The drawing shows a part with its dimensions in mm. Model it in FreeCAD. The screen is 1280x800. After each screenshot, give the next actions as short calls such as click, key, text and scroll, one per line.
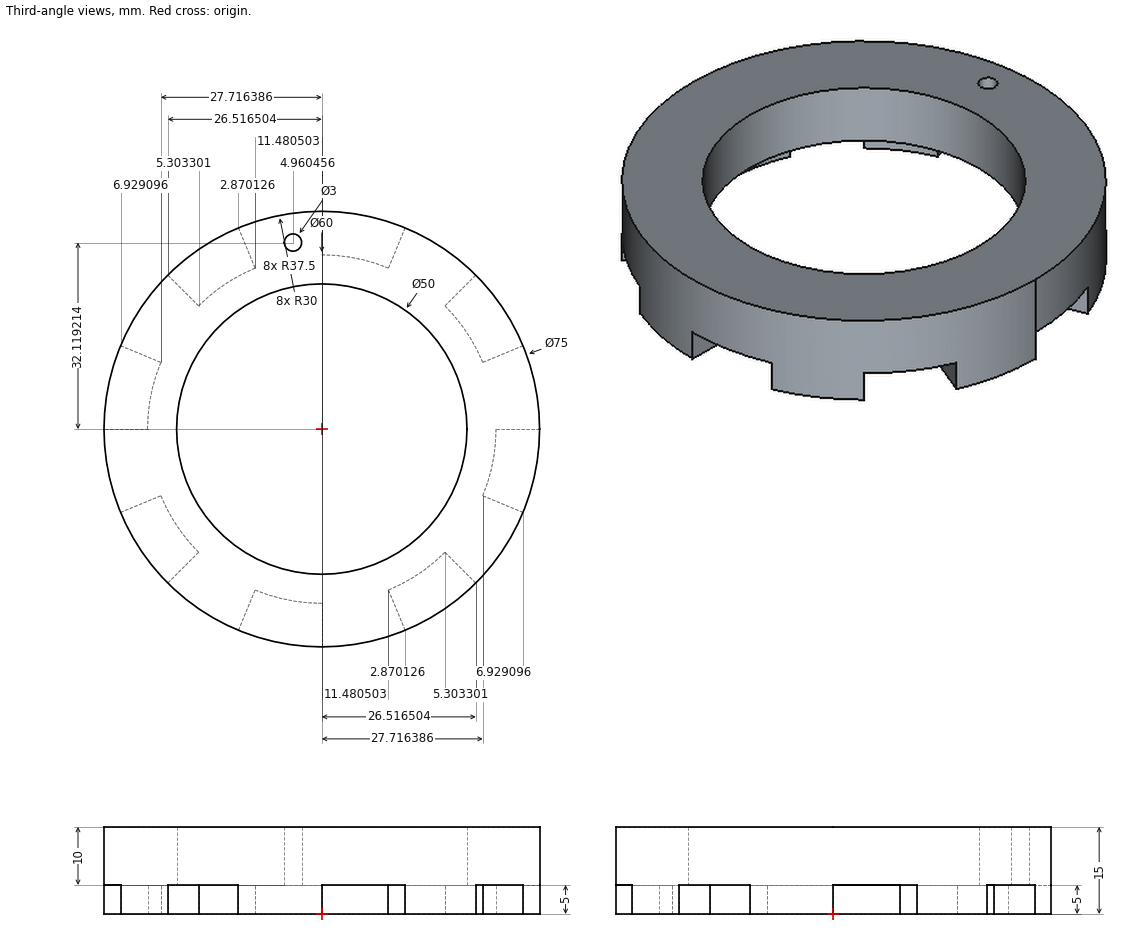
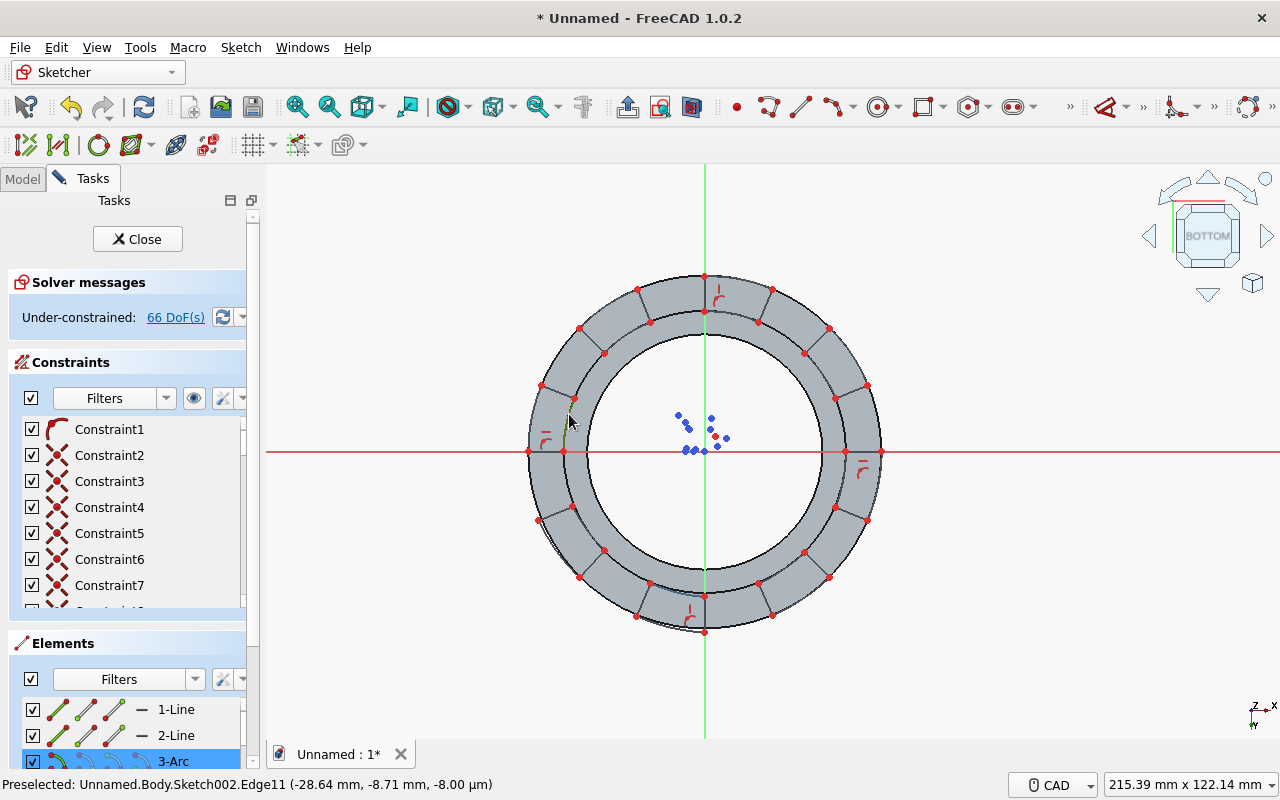
key(c)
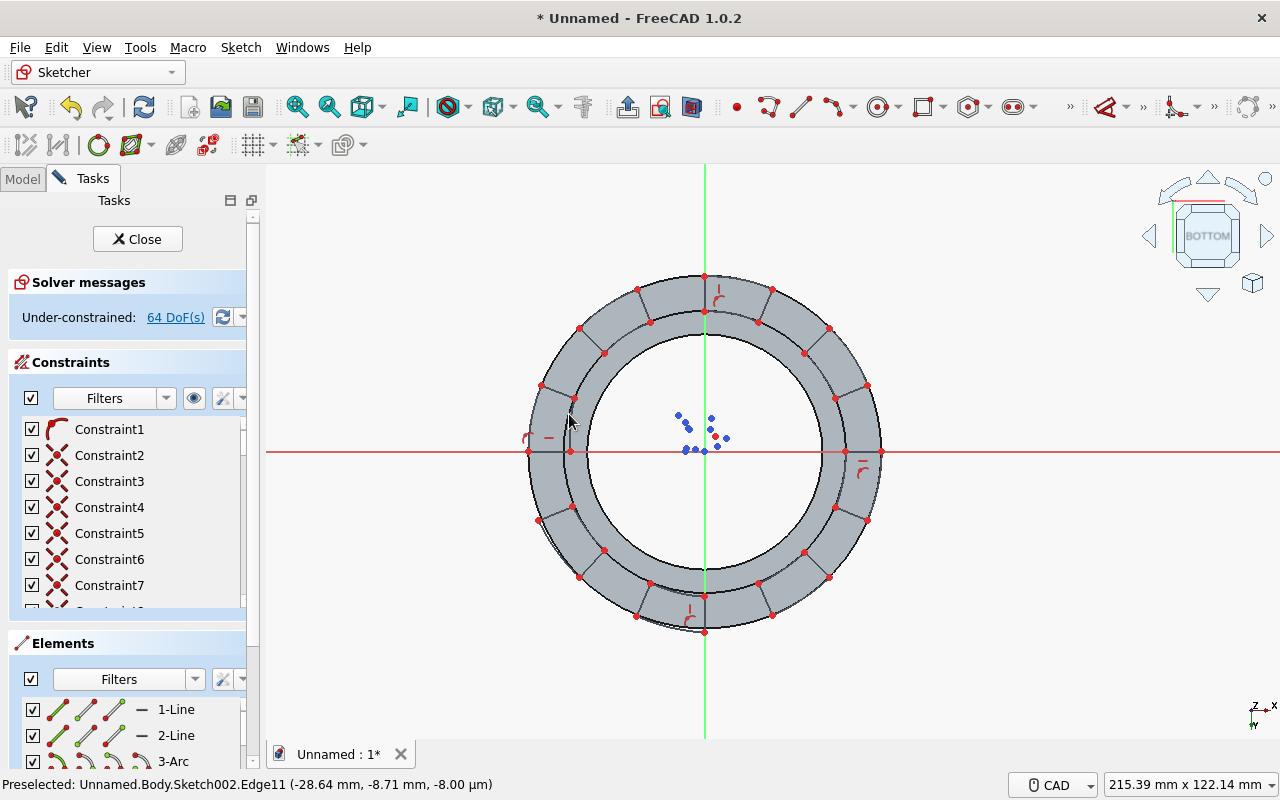
click(666, 589)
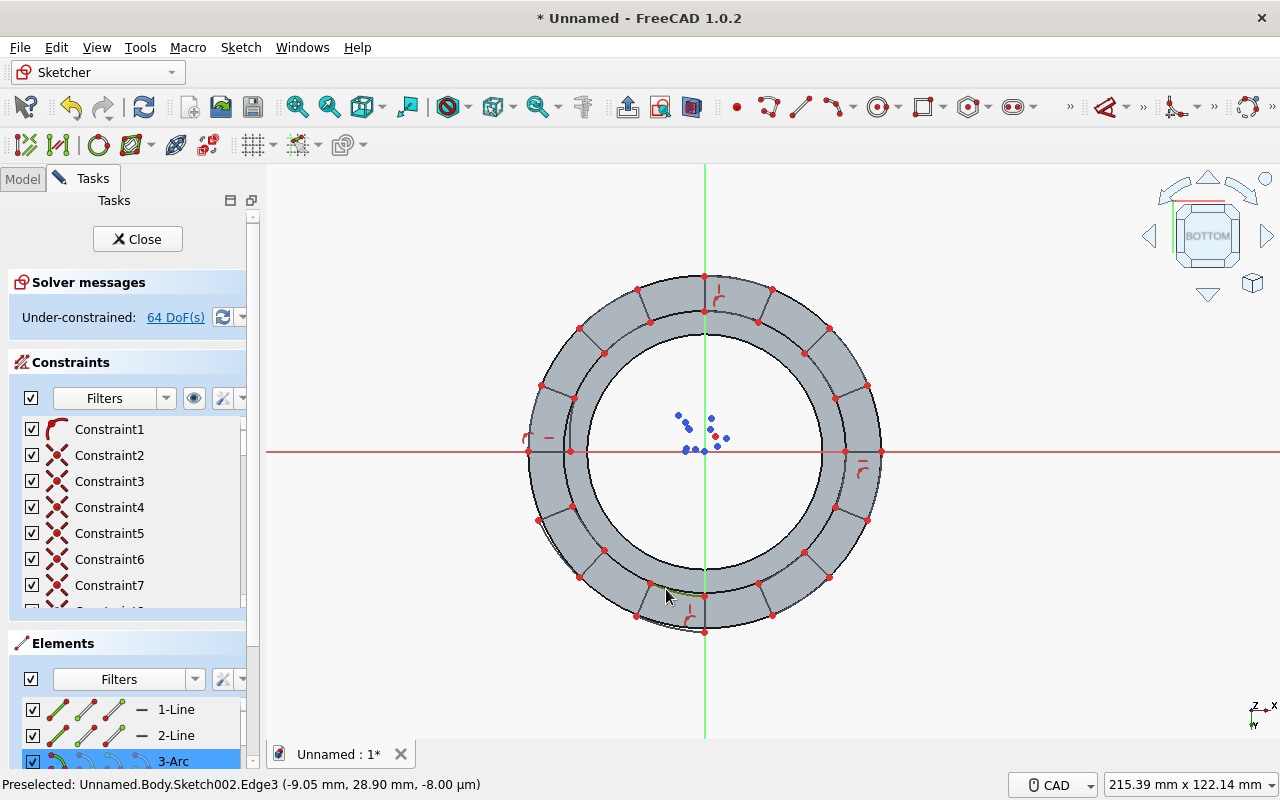
click(535, 405)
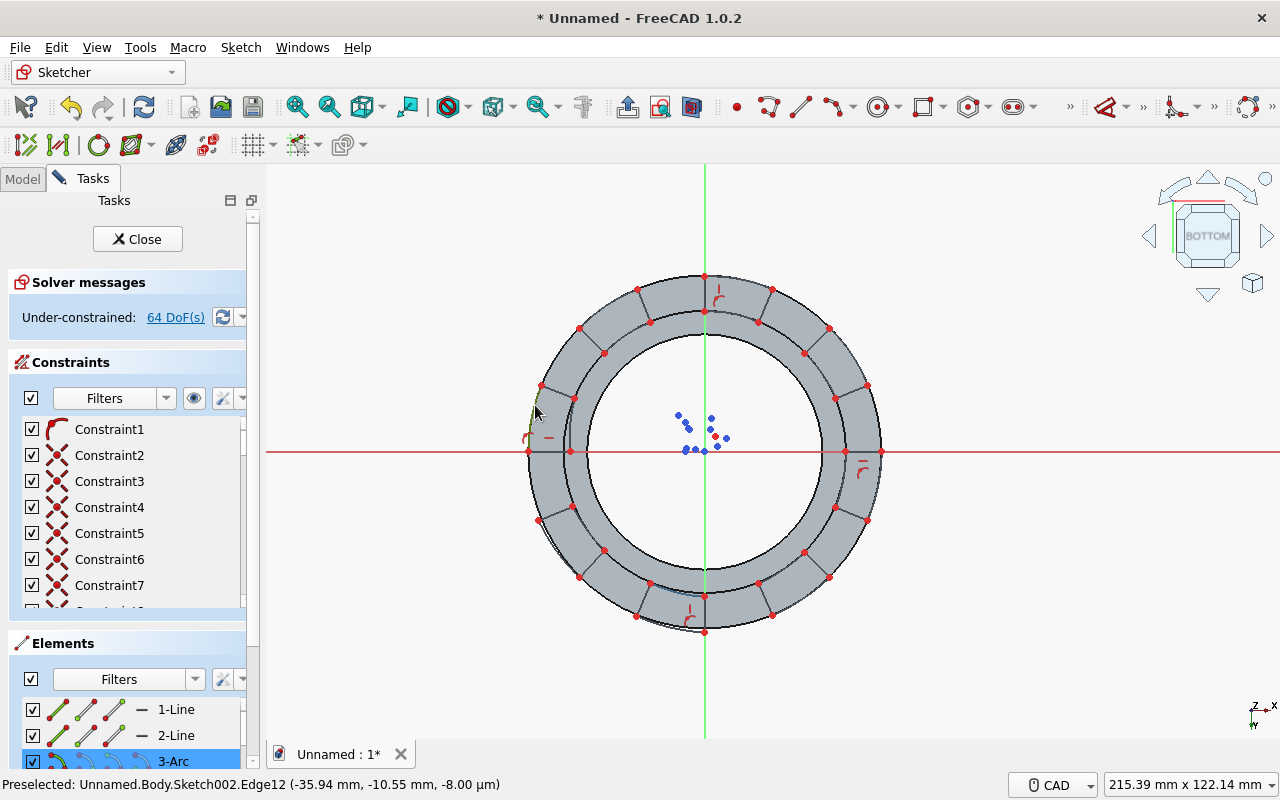
key(c)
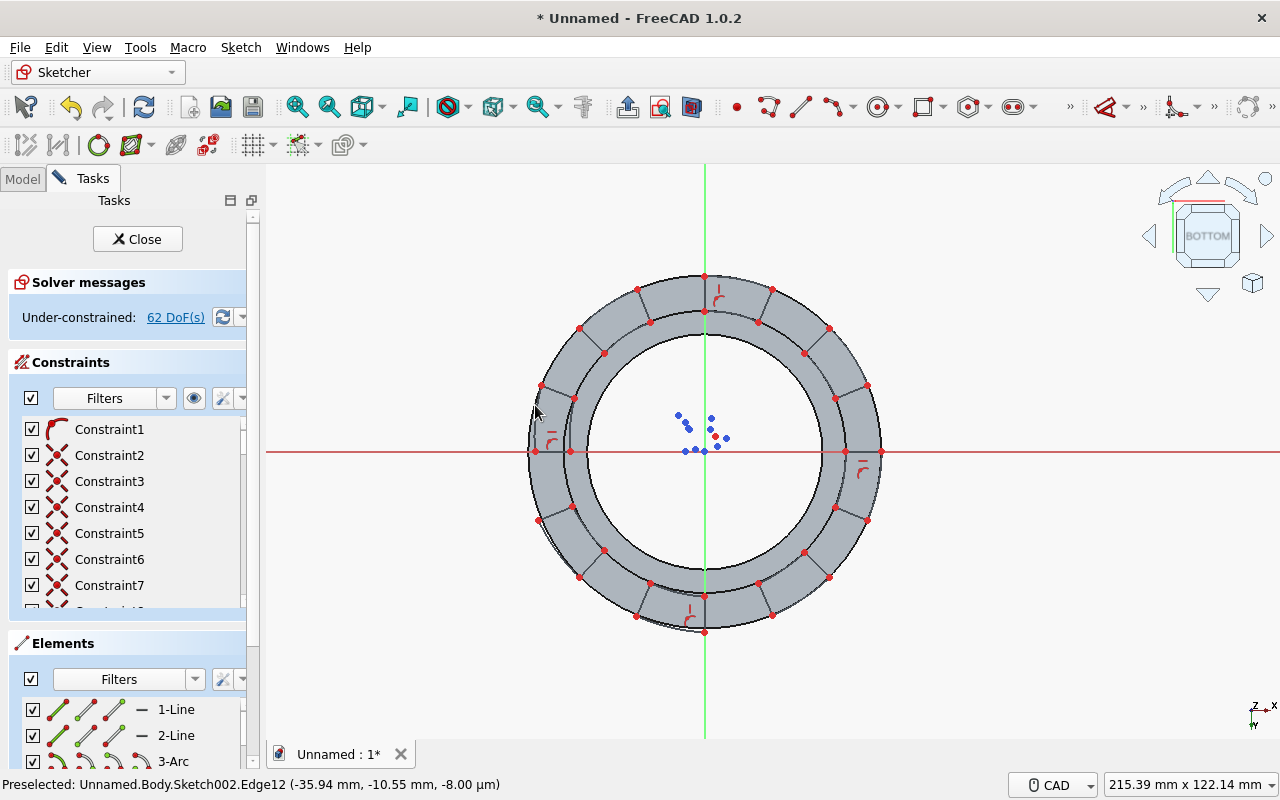
click(666, 589)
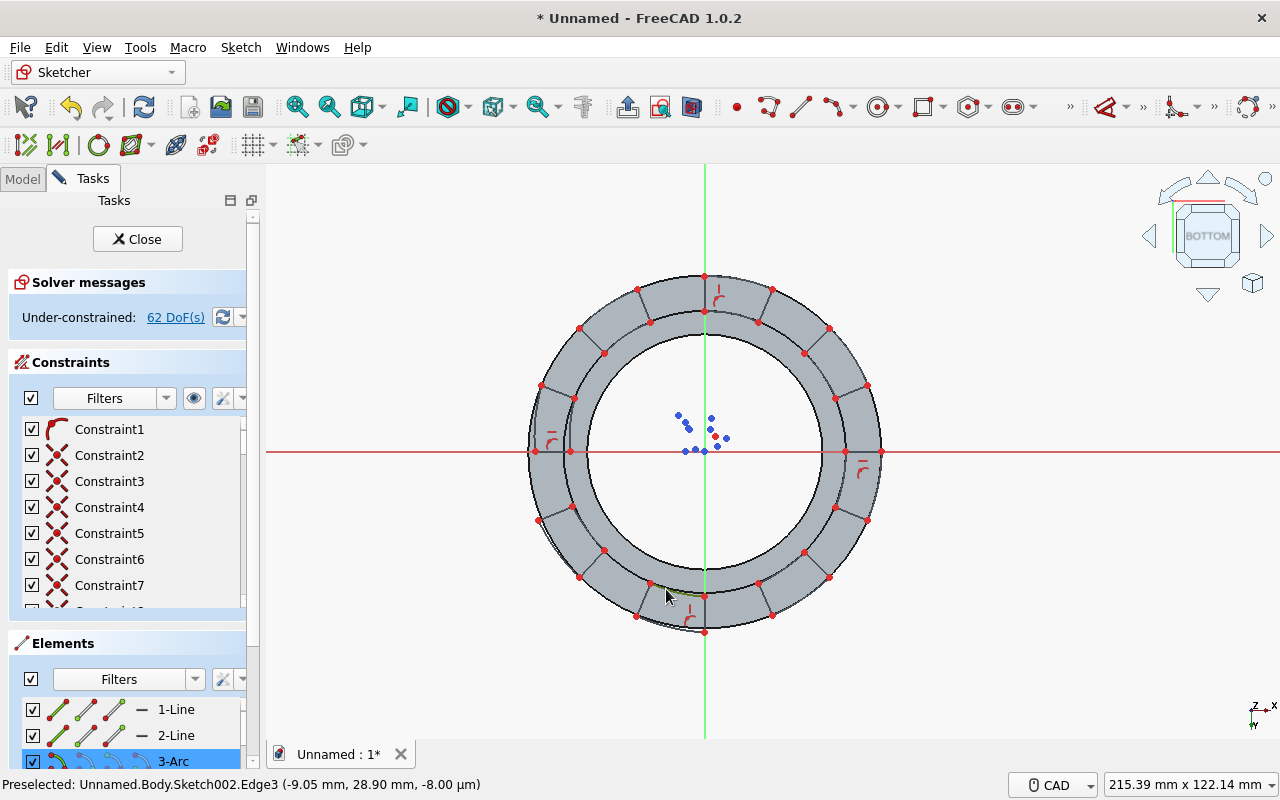
click(635, 329)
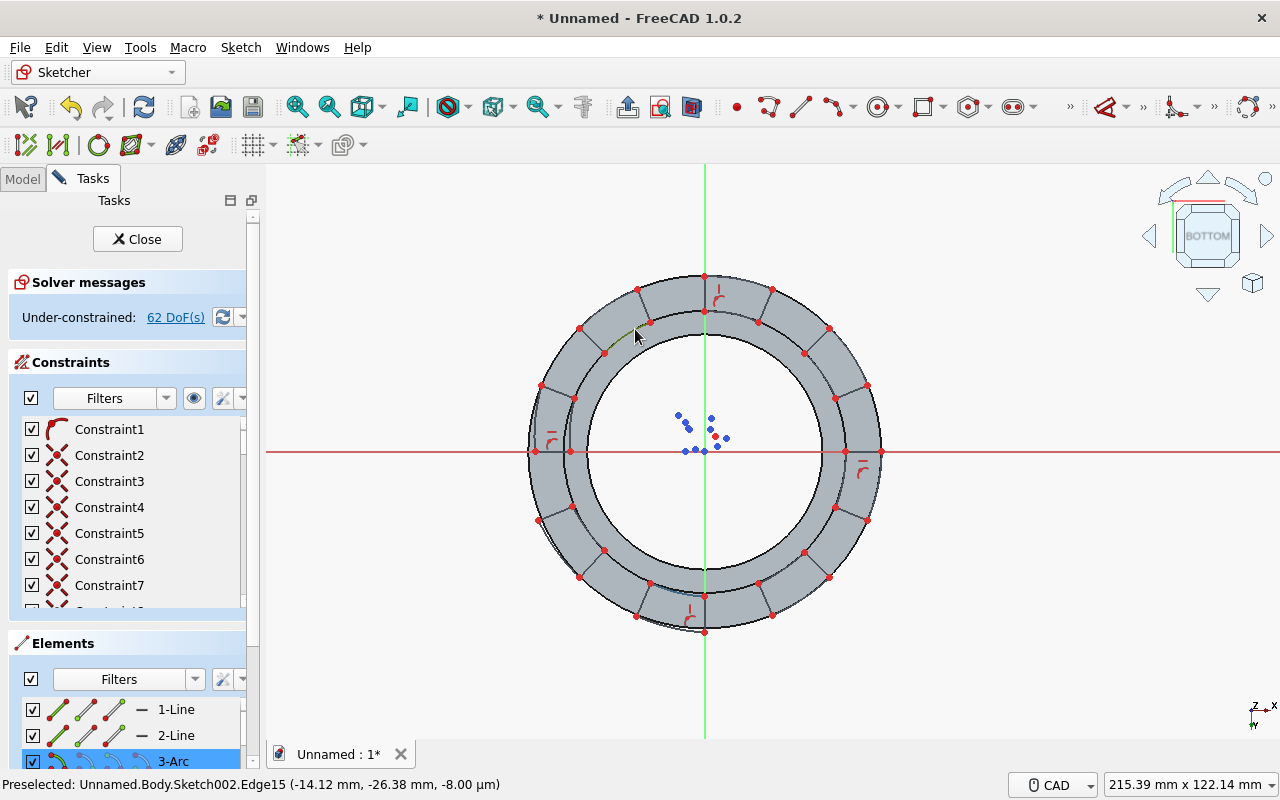
key(c)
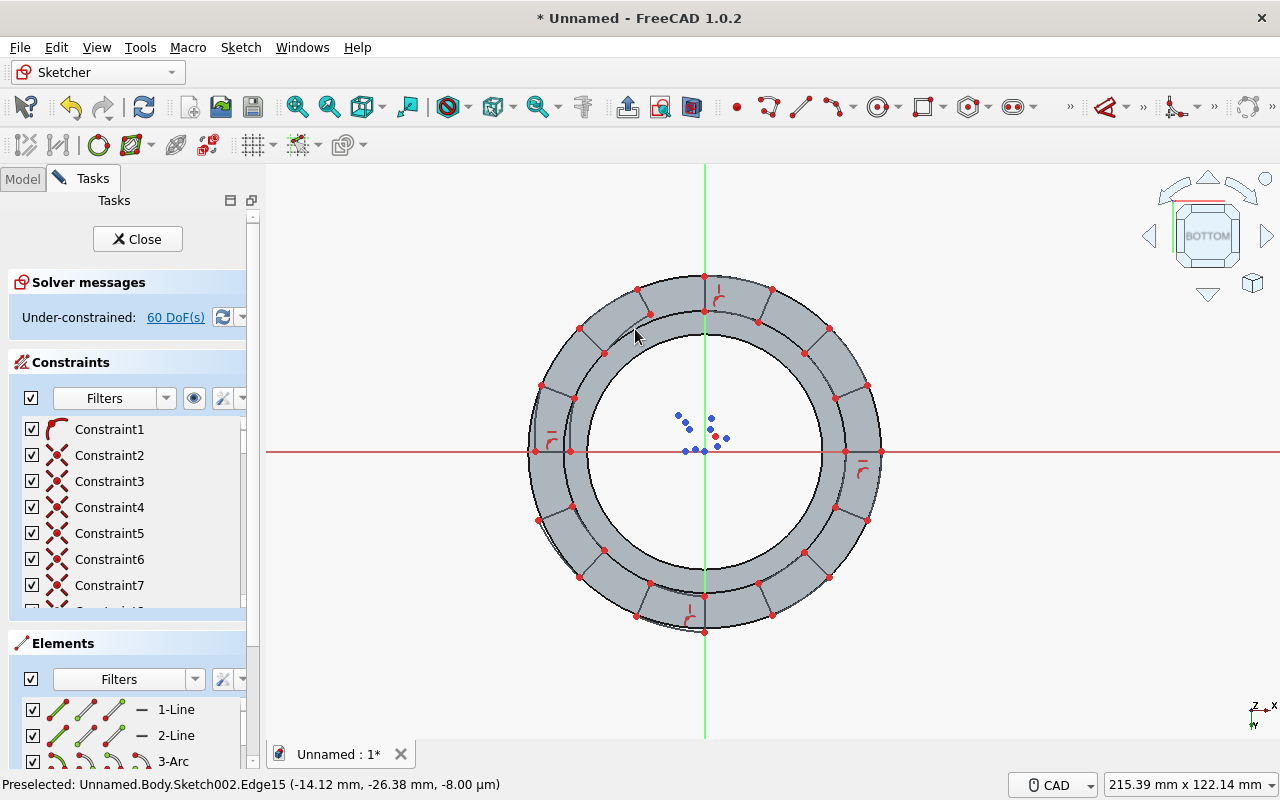
click(666, 589)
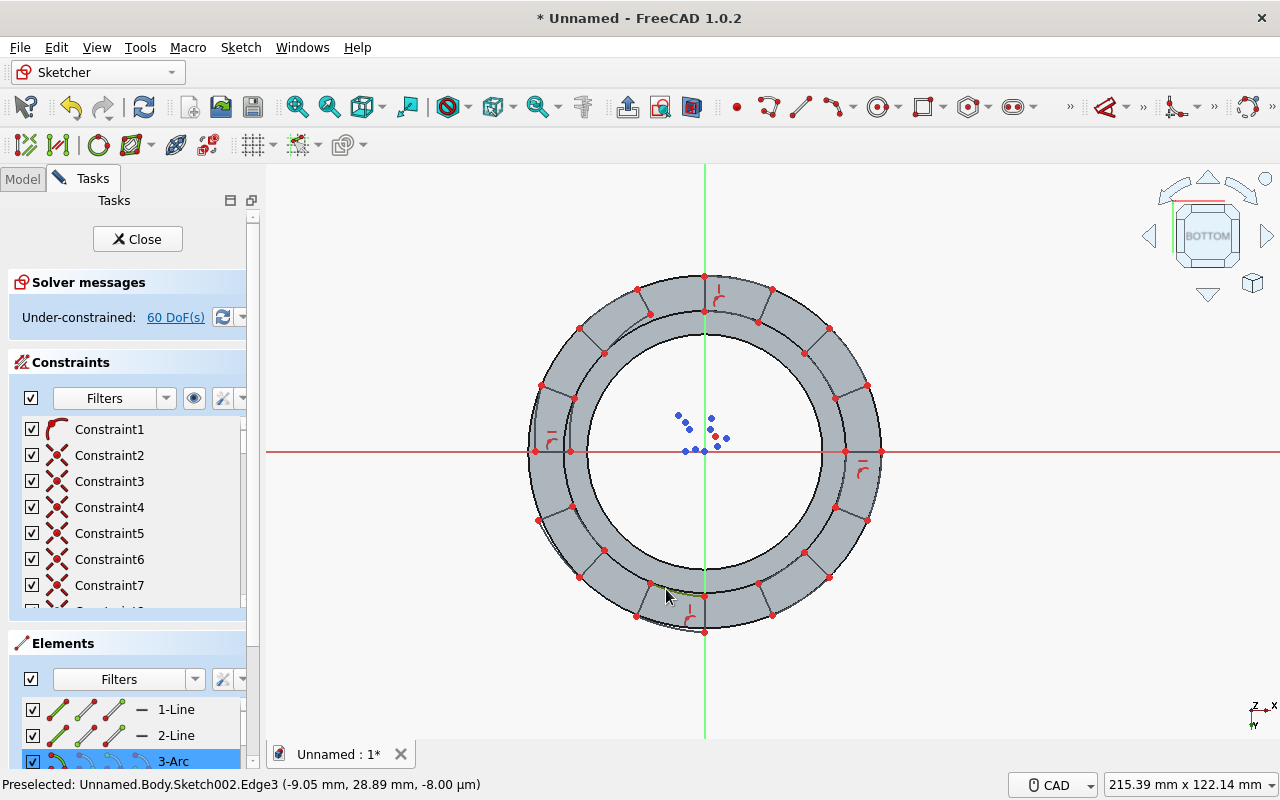
click(618, 298)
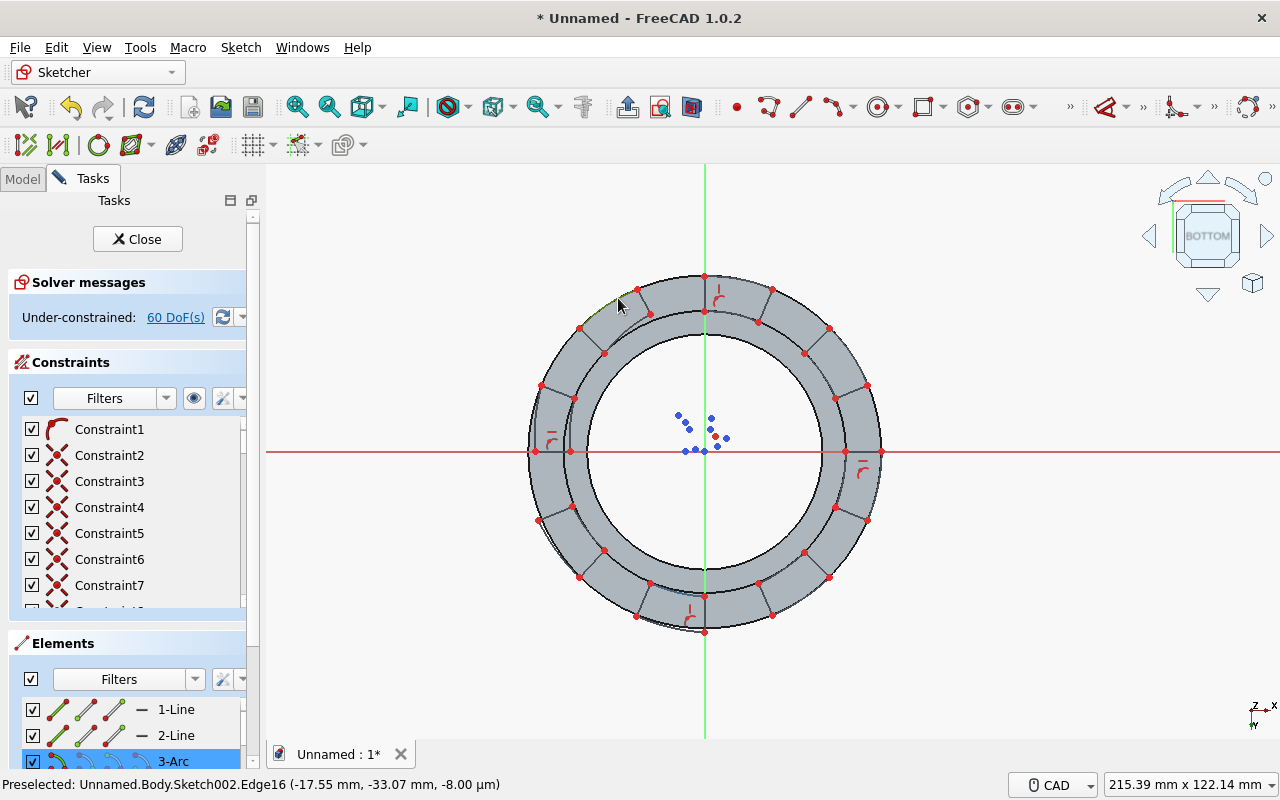
key(c)